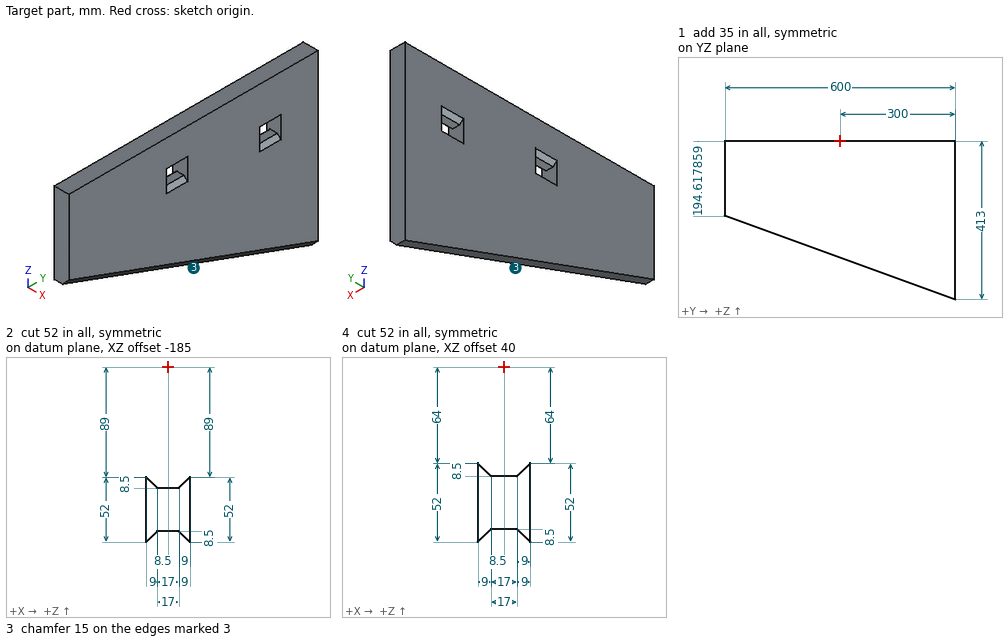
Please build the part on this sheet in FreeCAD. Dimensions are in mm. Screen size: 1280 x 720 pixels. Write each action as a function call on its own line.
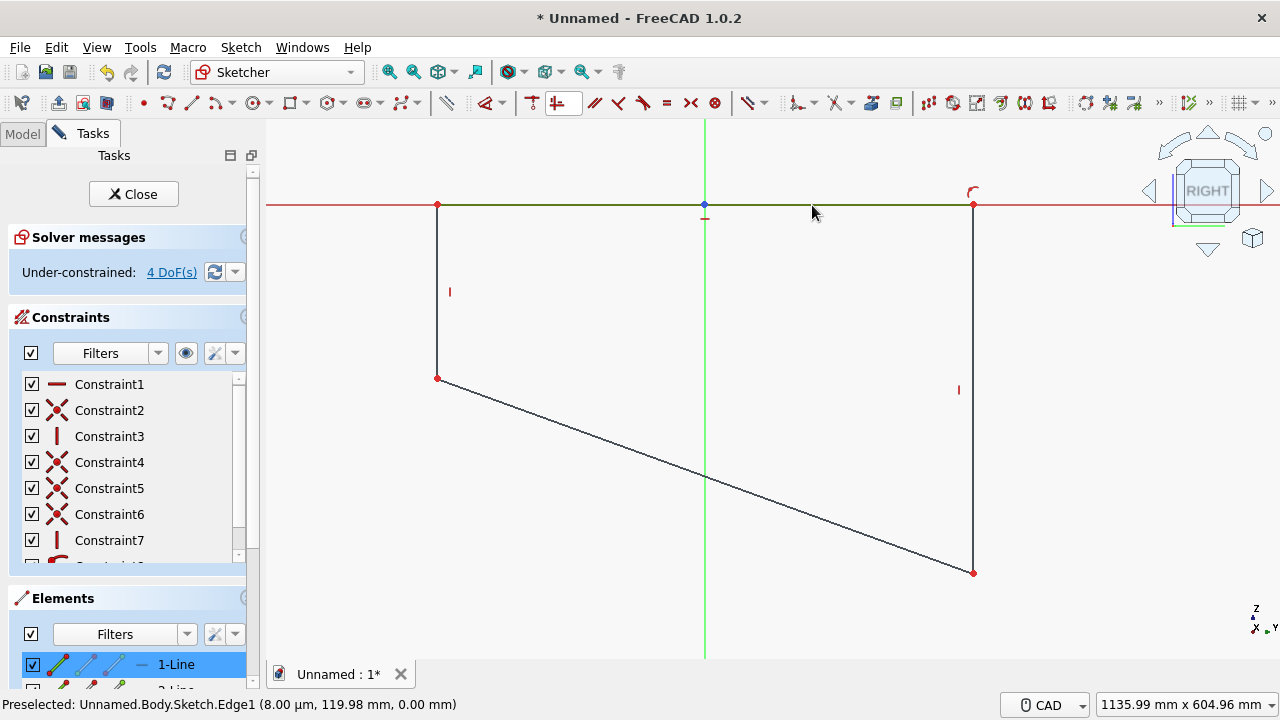
key(l)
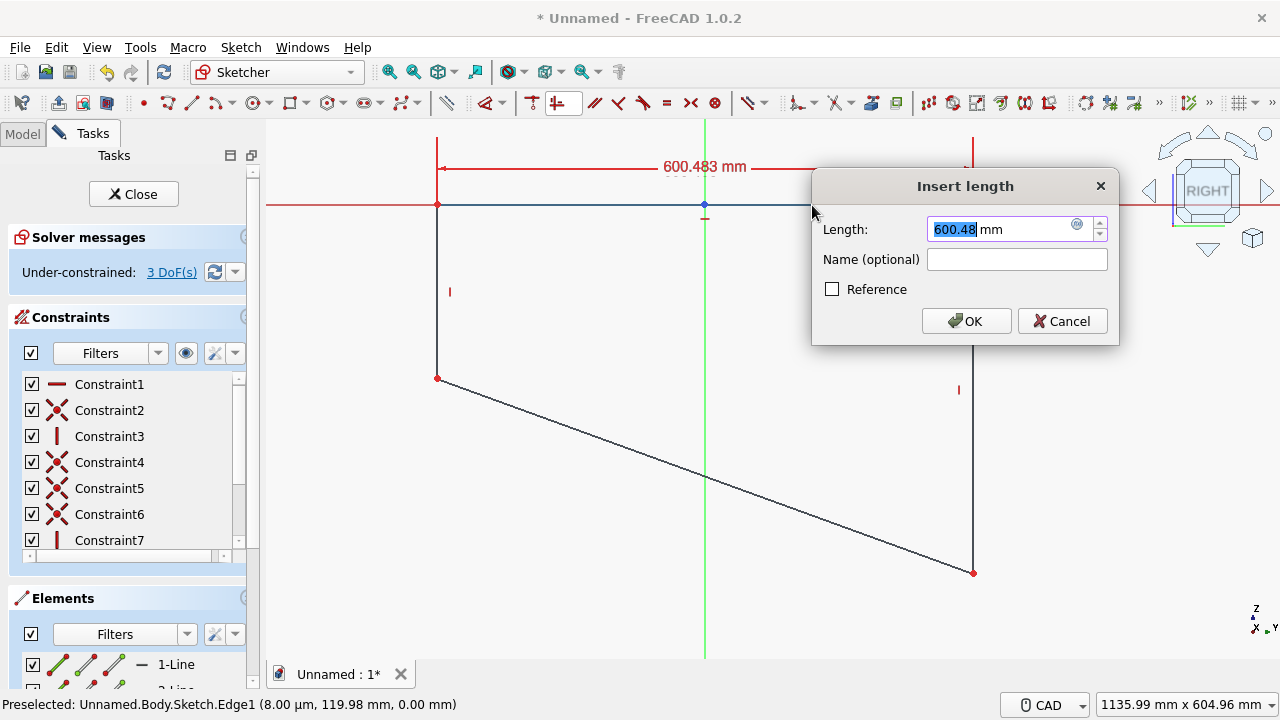
text(600)
key(Return)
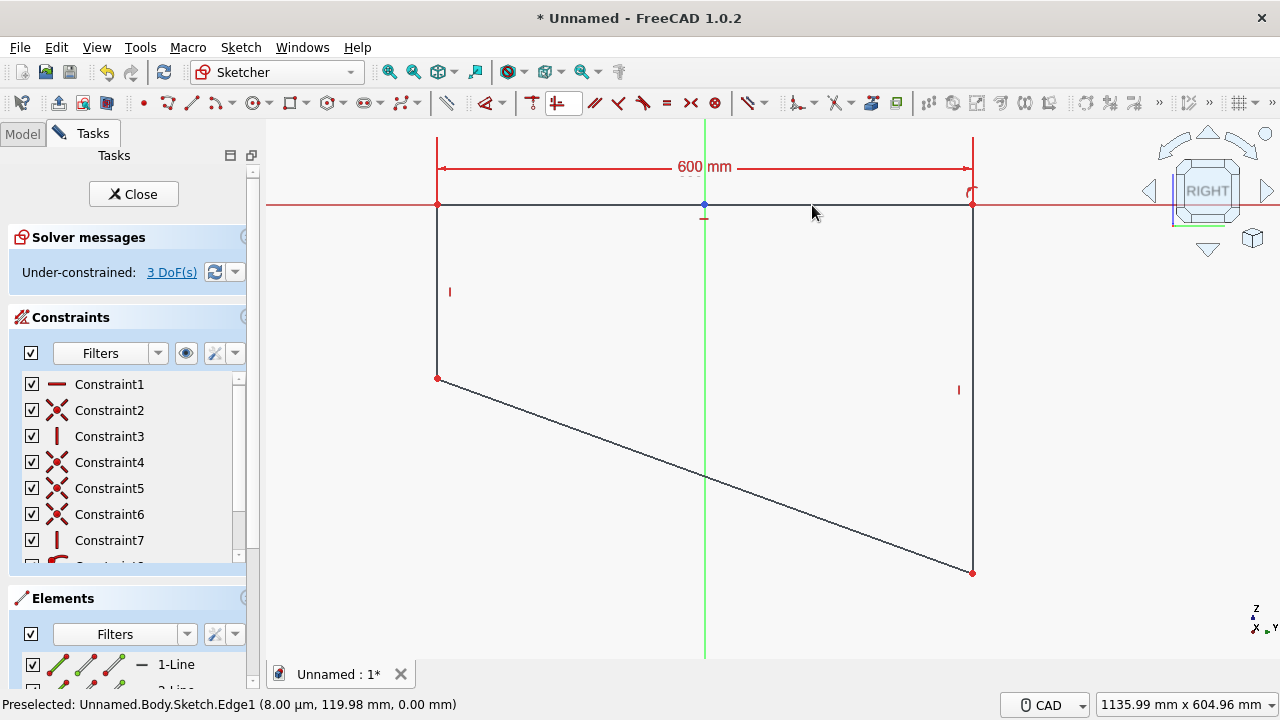
click(973, 463)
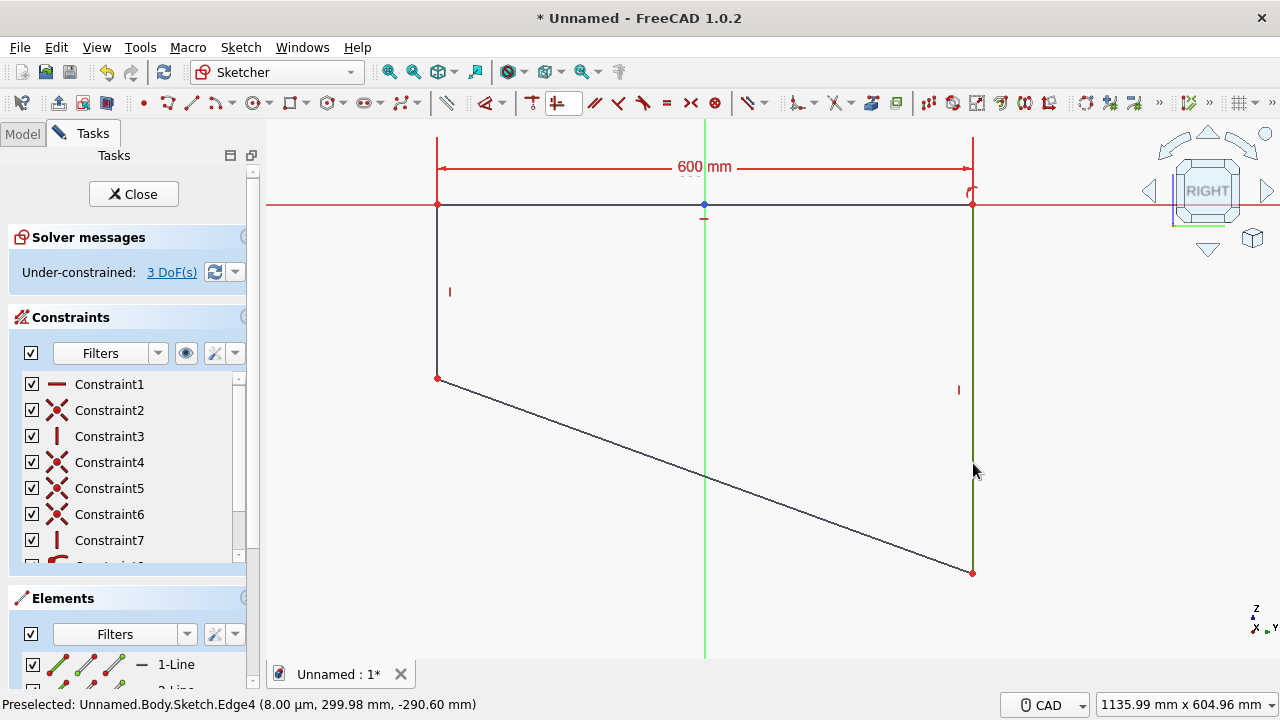
key(i)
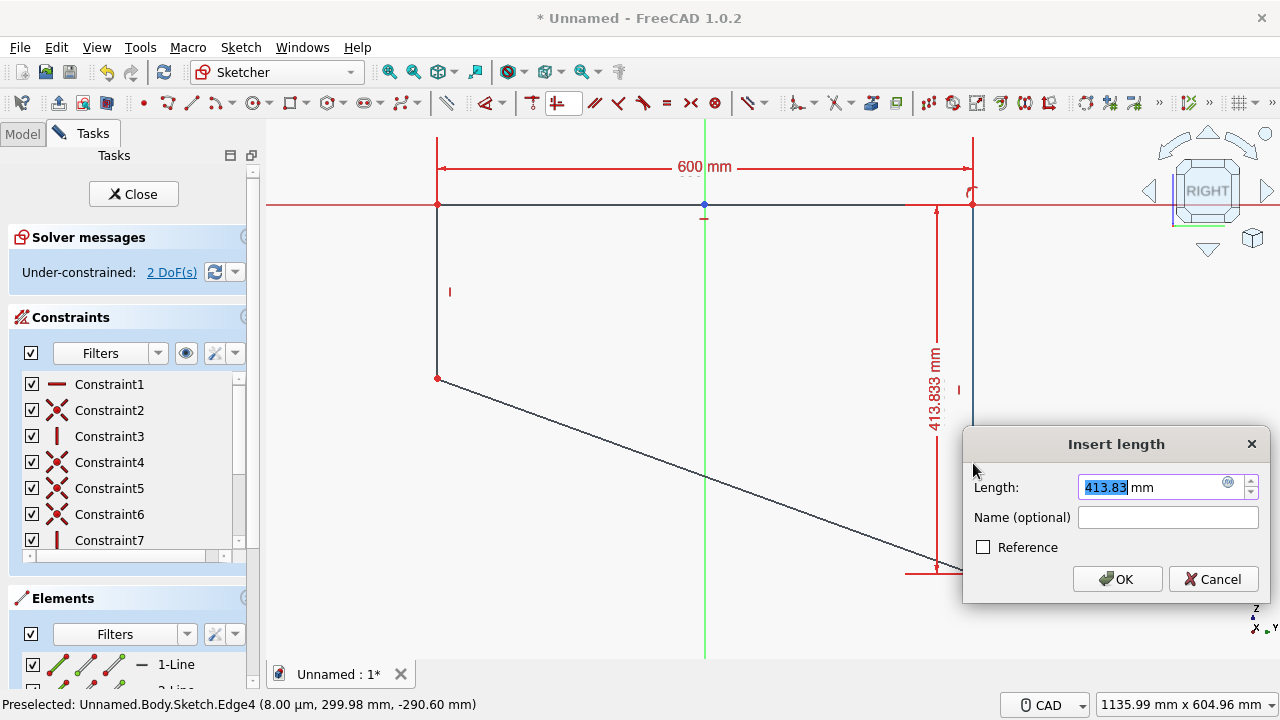
text(413)
key(Return)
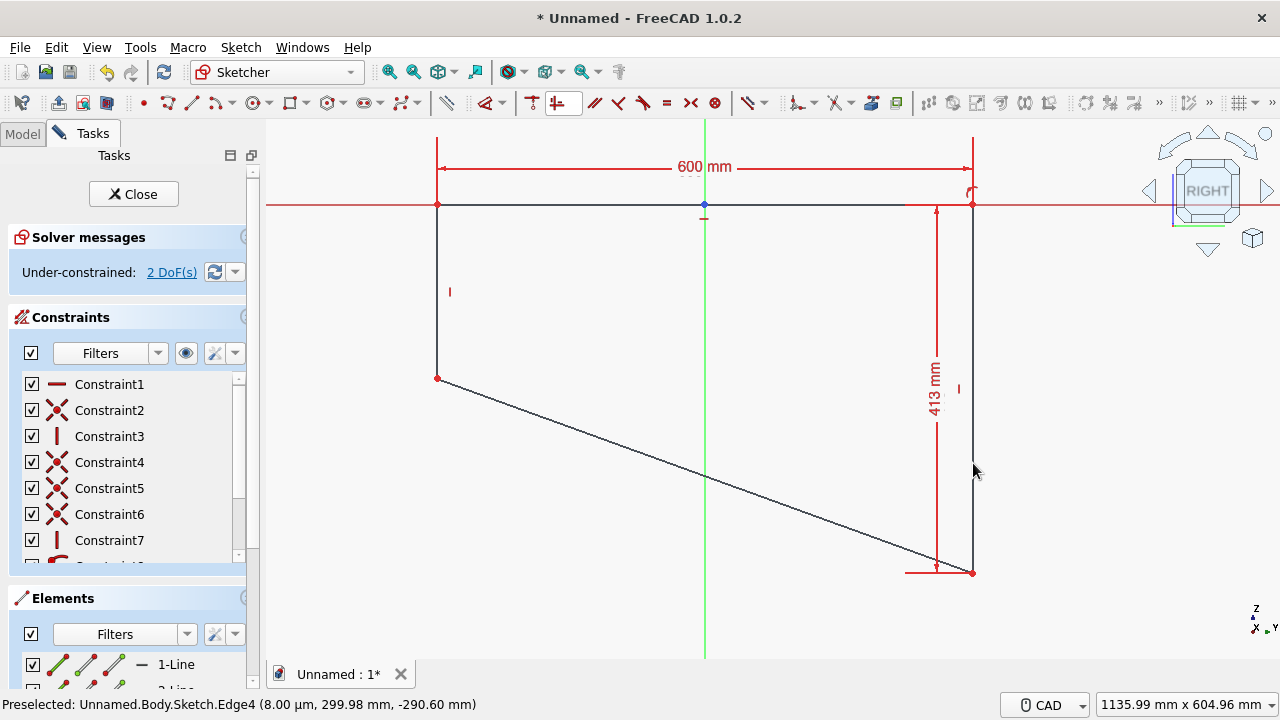
click(973, 205)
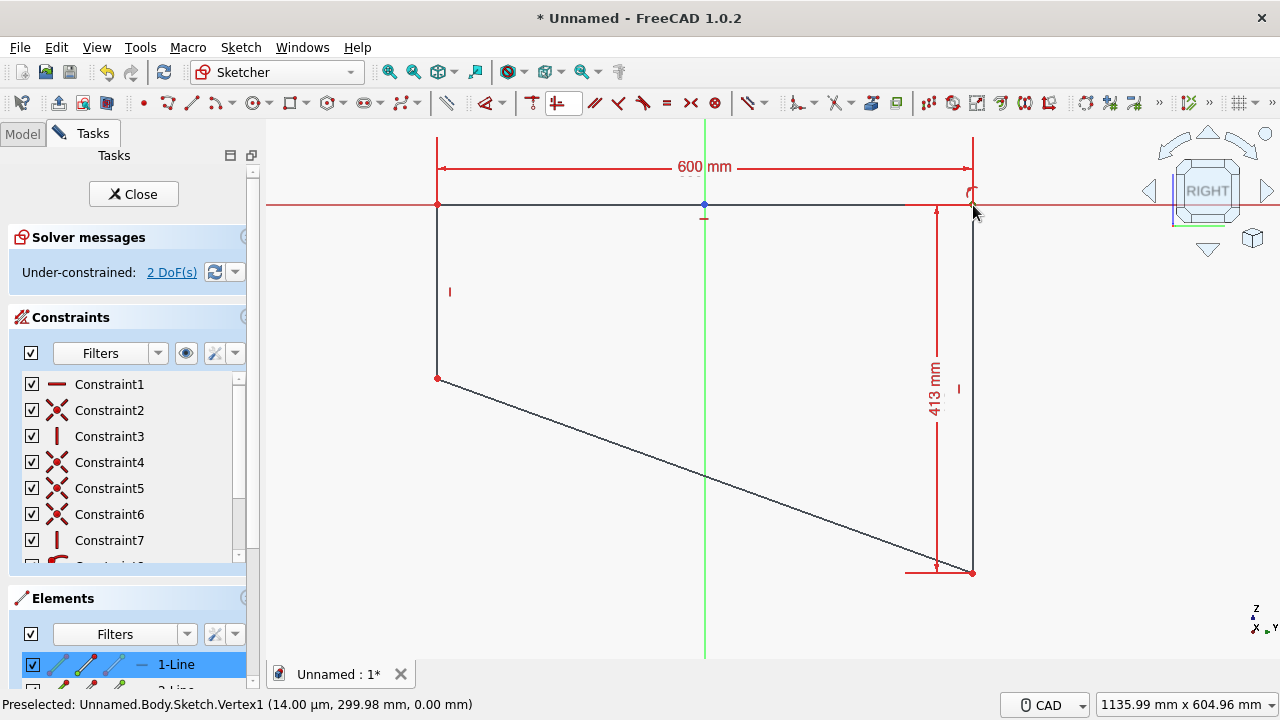
key(l)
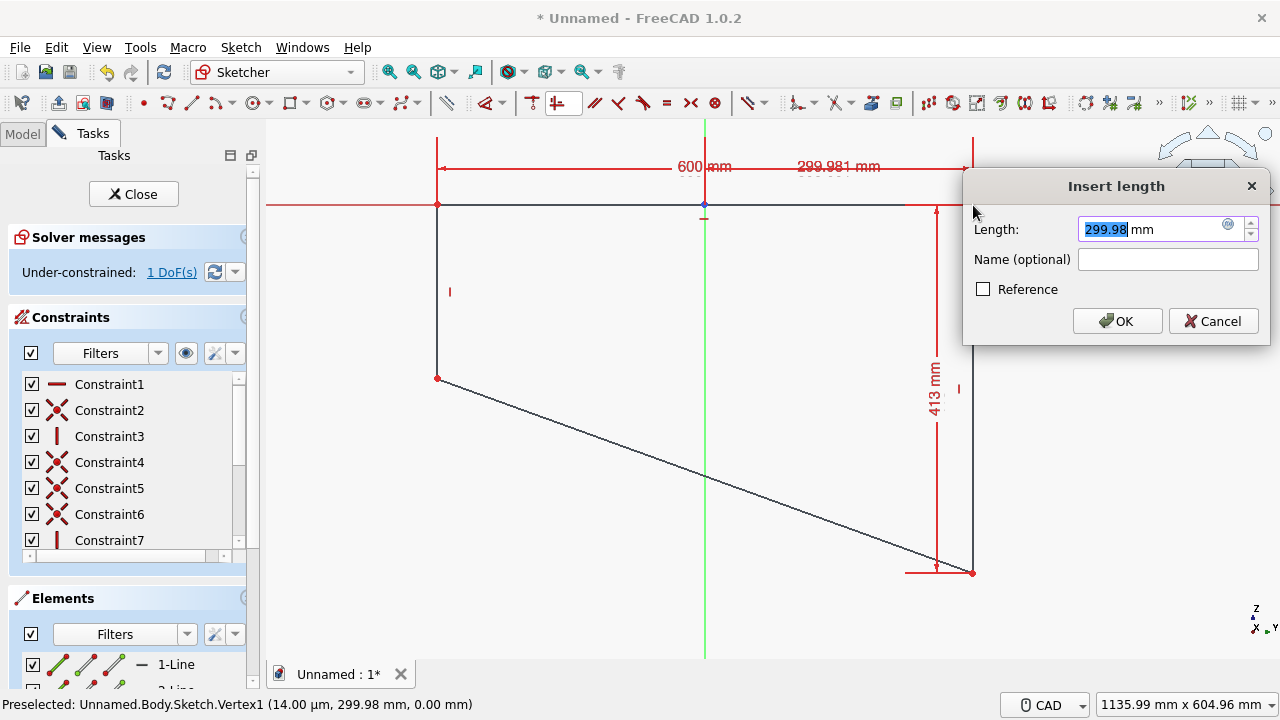
text(300)
key(Return)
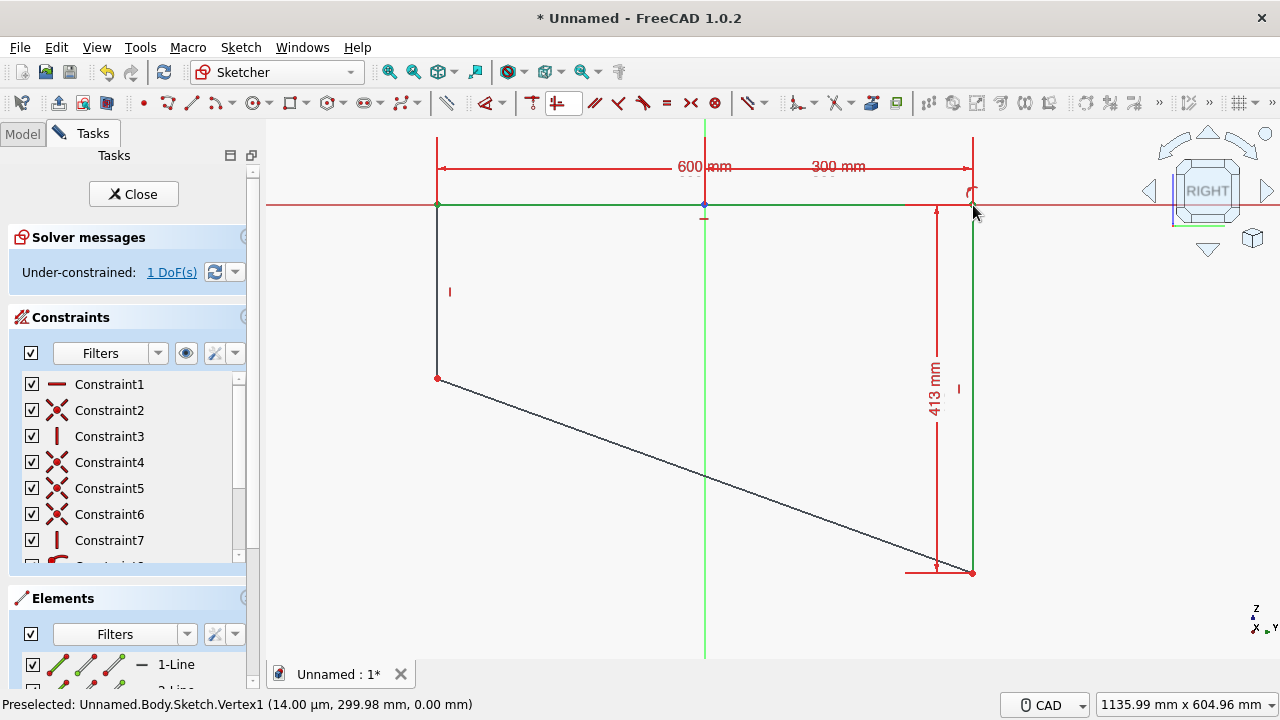
click(437, 257)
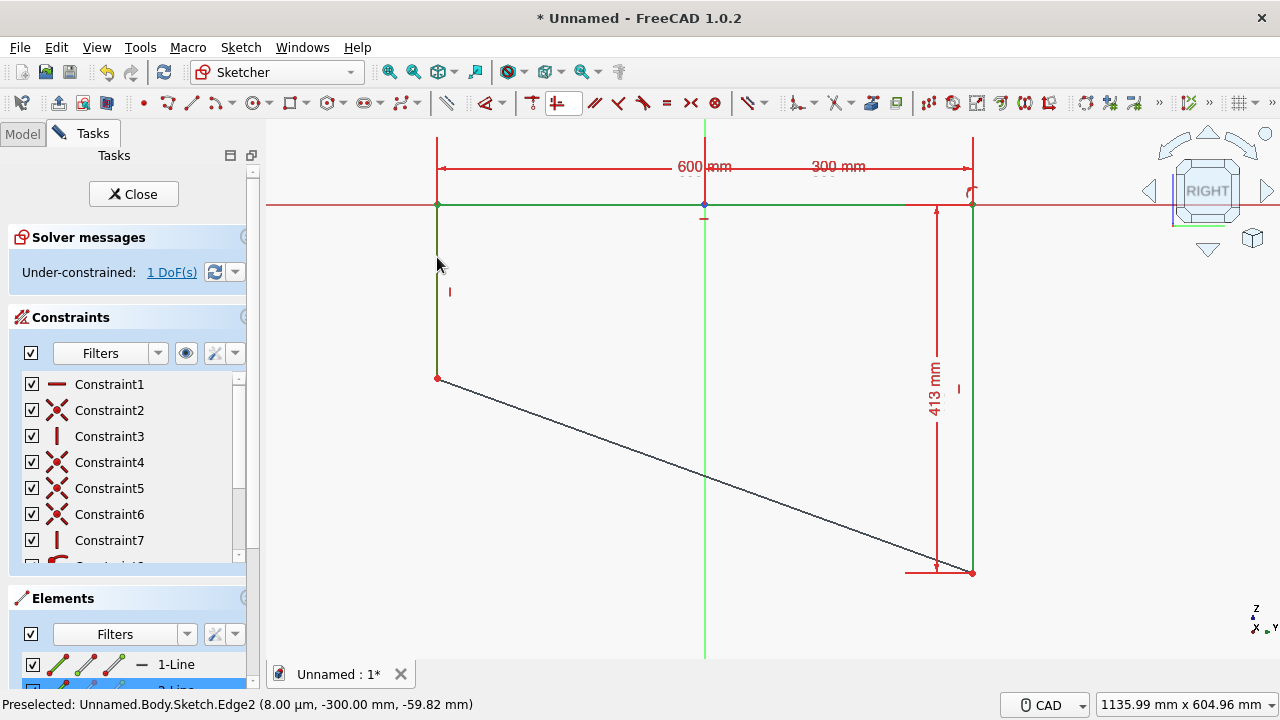
key(i)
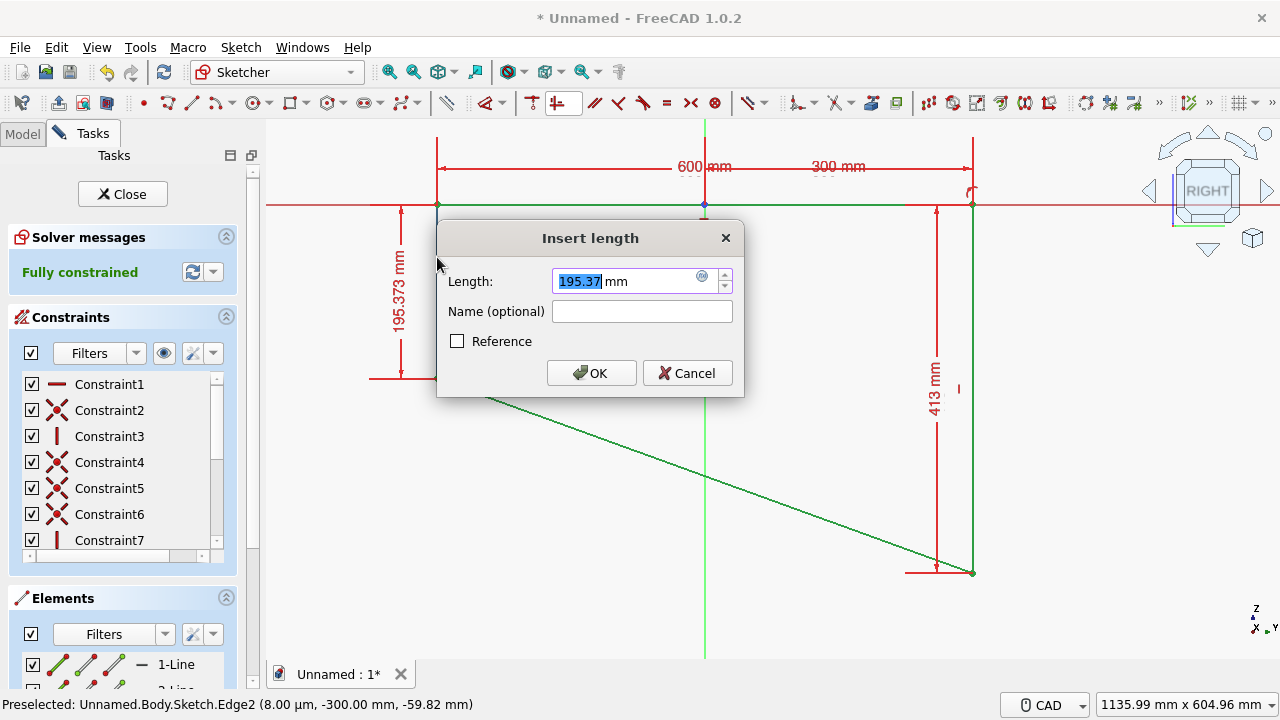
text(194.617859)
key(Return)